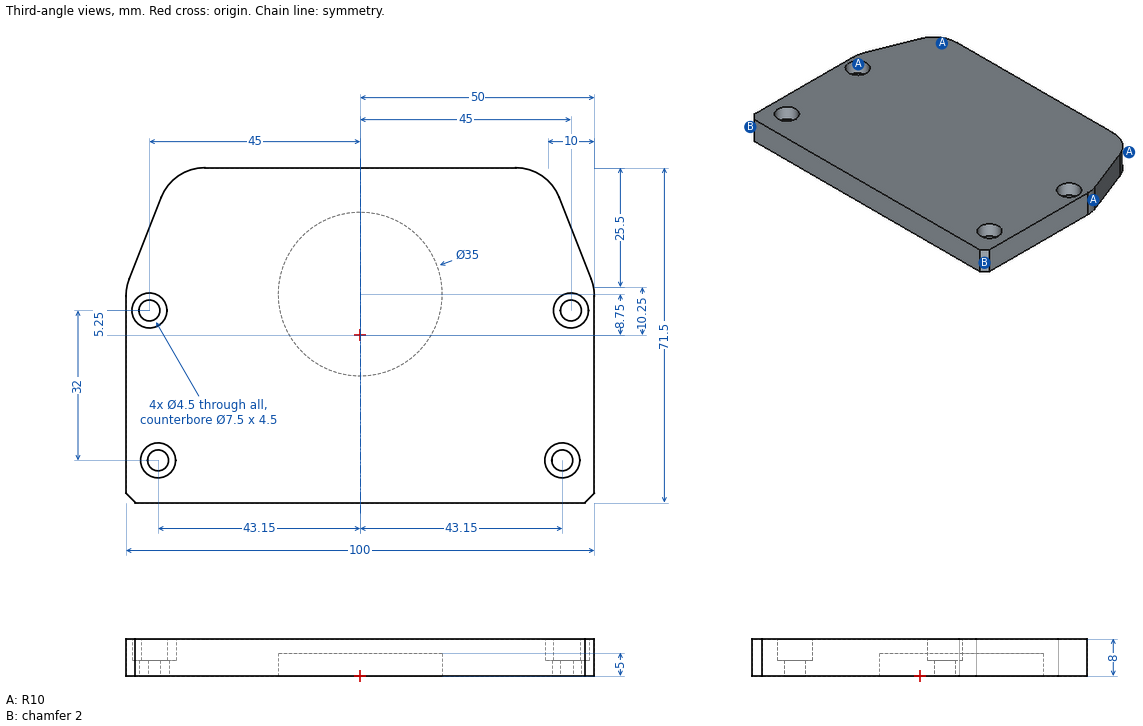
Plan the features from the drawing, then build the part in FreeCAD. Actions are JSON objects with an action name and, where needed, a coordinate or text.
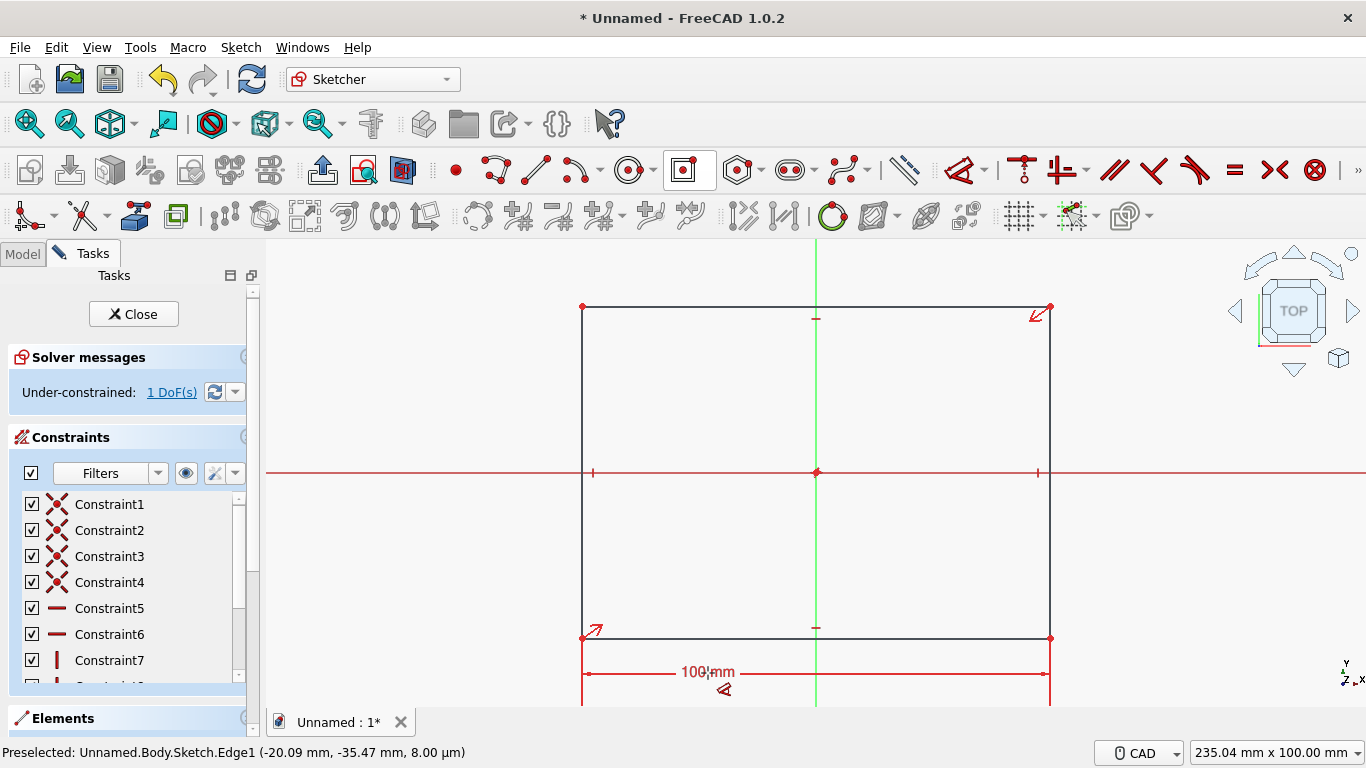
{"action": "left_click", "coordinate": [1050, 539]}
{"action": "left_click", "coordinate": [1084, 397]}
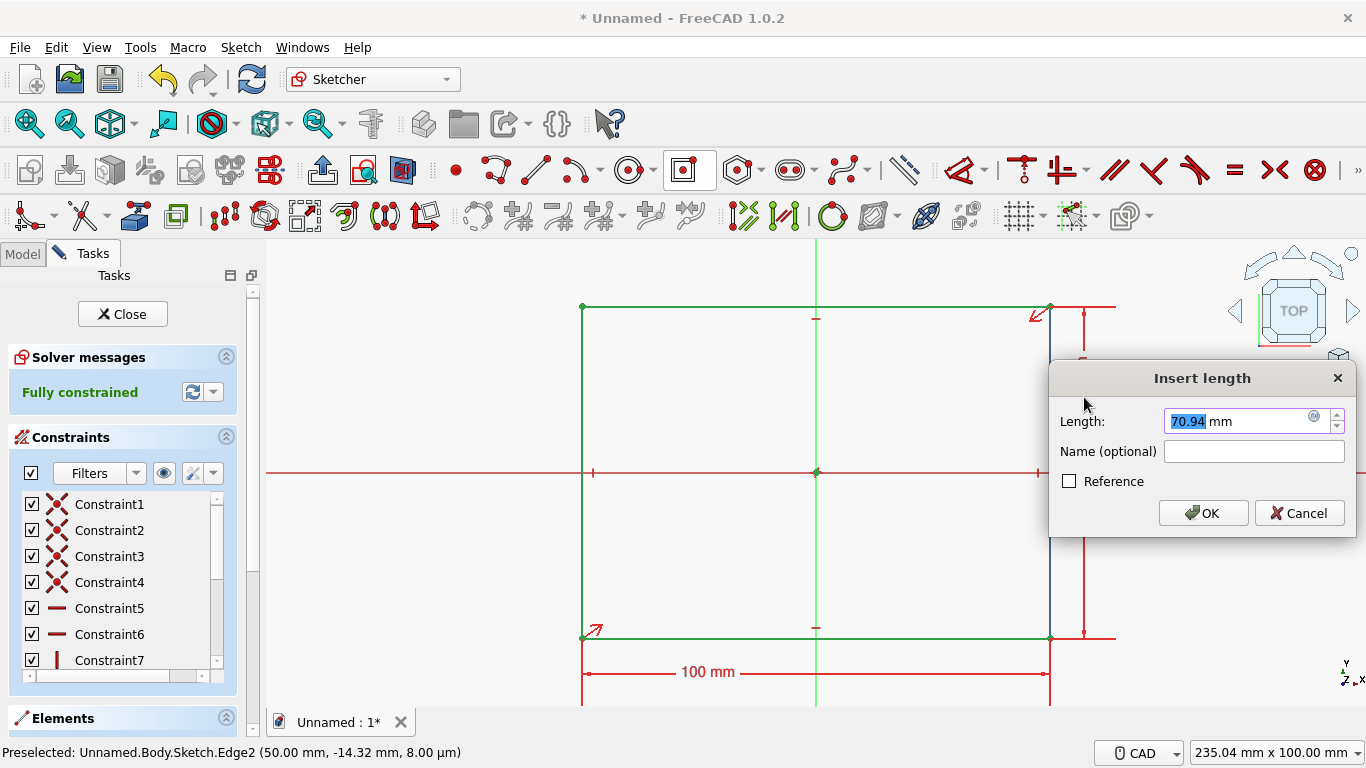
{"action": "type", "text": "71.5"}
{"action": "key", "text": "Return"}
{"action": "key", "text": "Escape"}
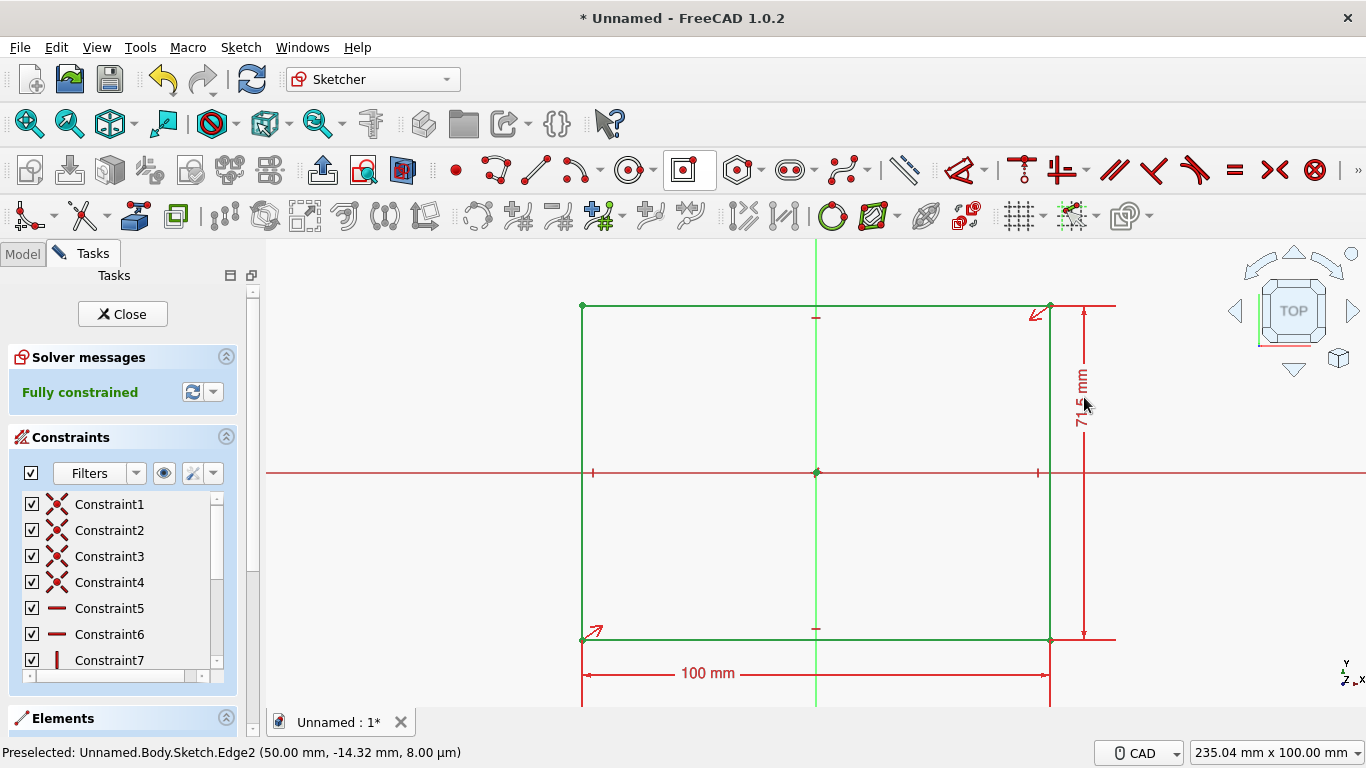
{"action": "left_click", "coordinate": [123, 314]}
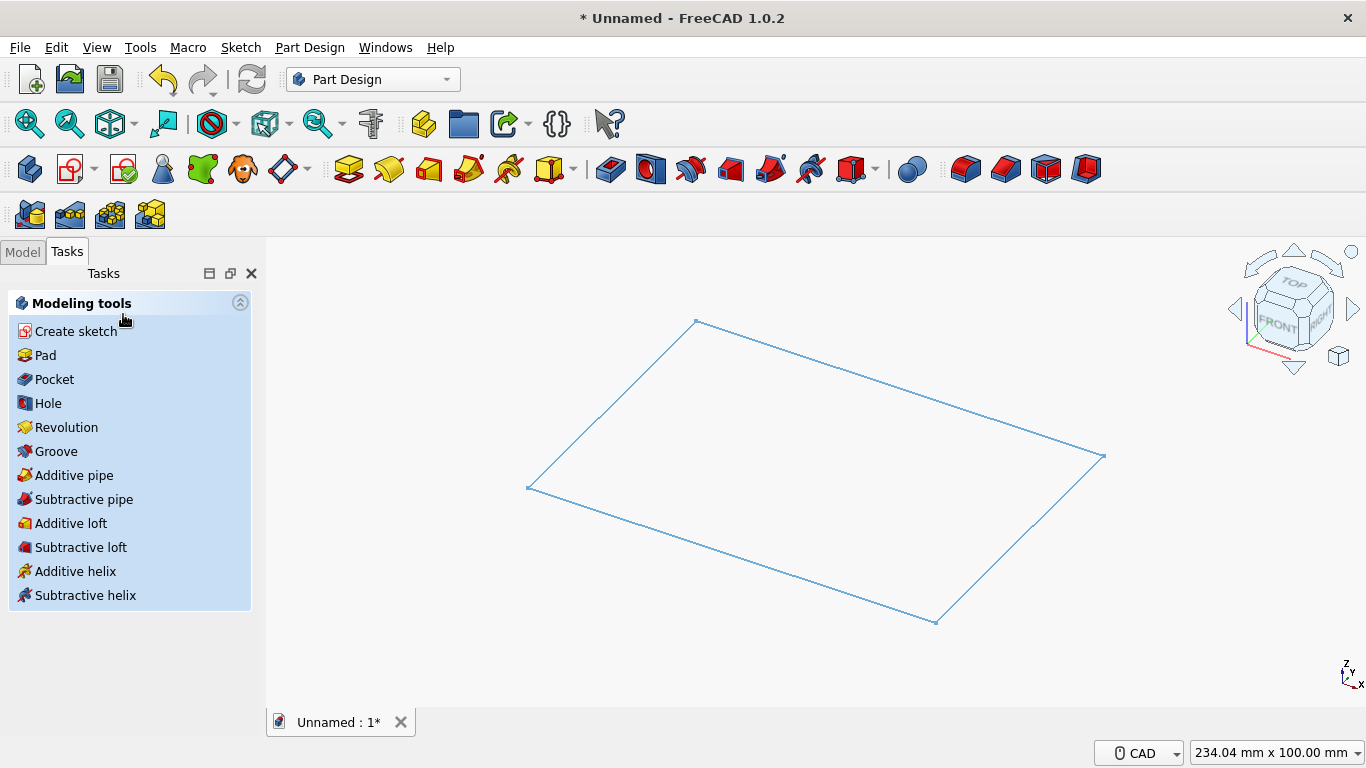
{"action": "left_click", "coordinate": [350, 170]}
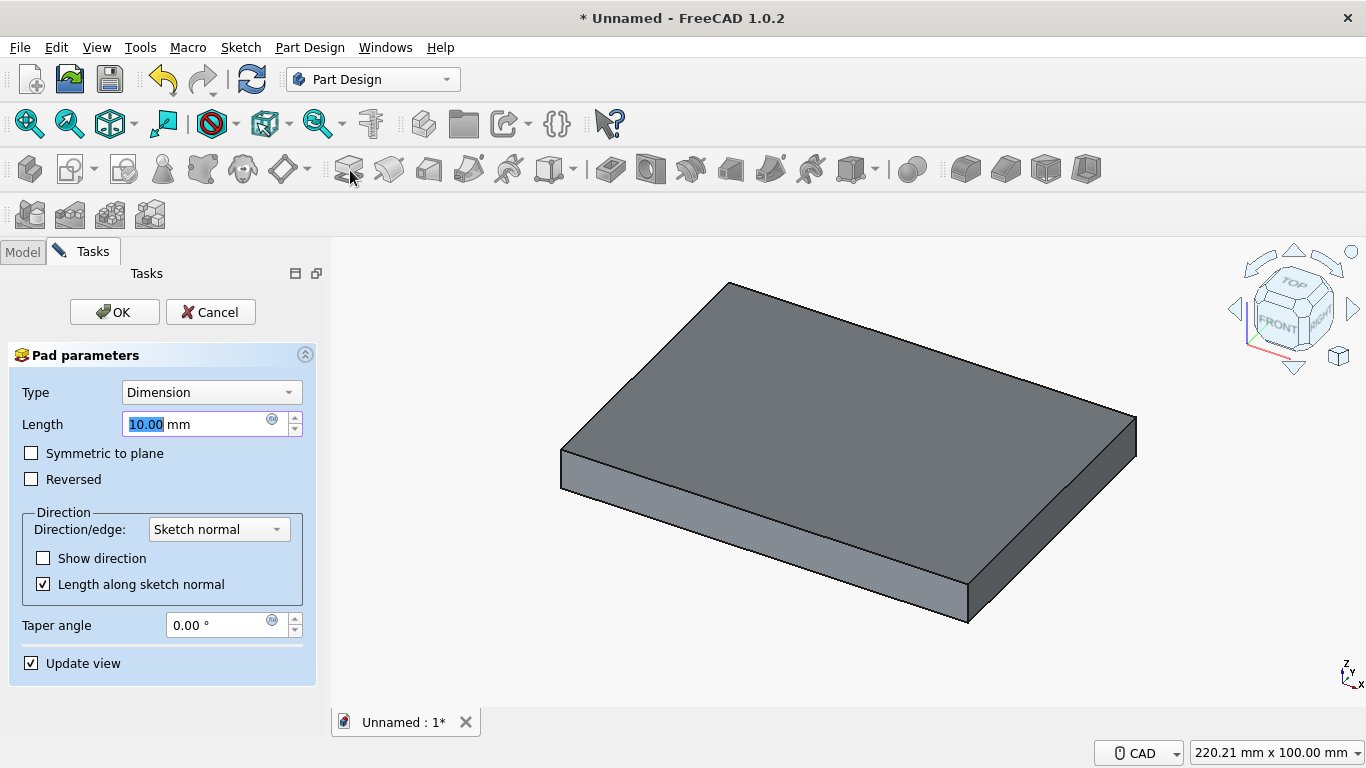
{"action": "type", "text": "8"}
{"action": "key", "text": "Tab"}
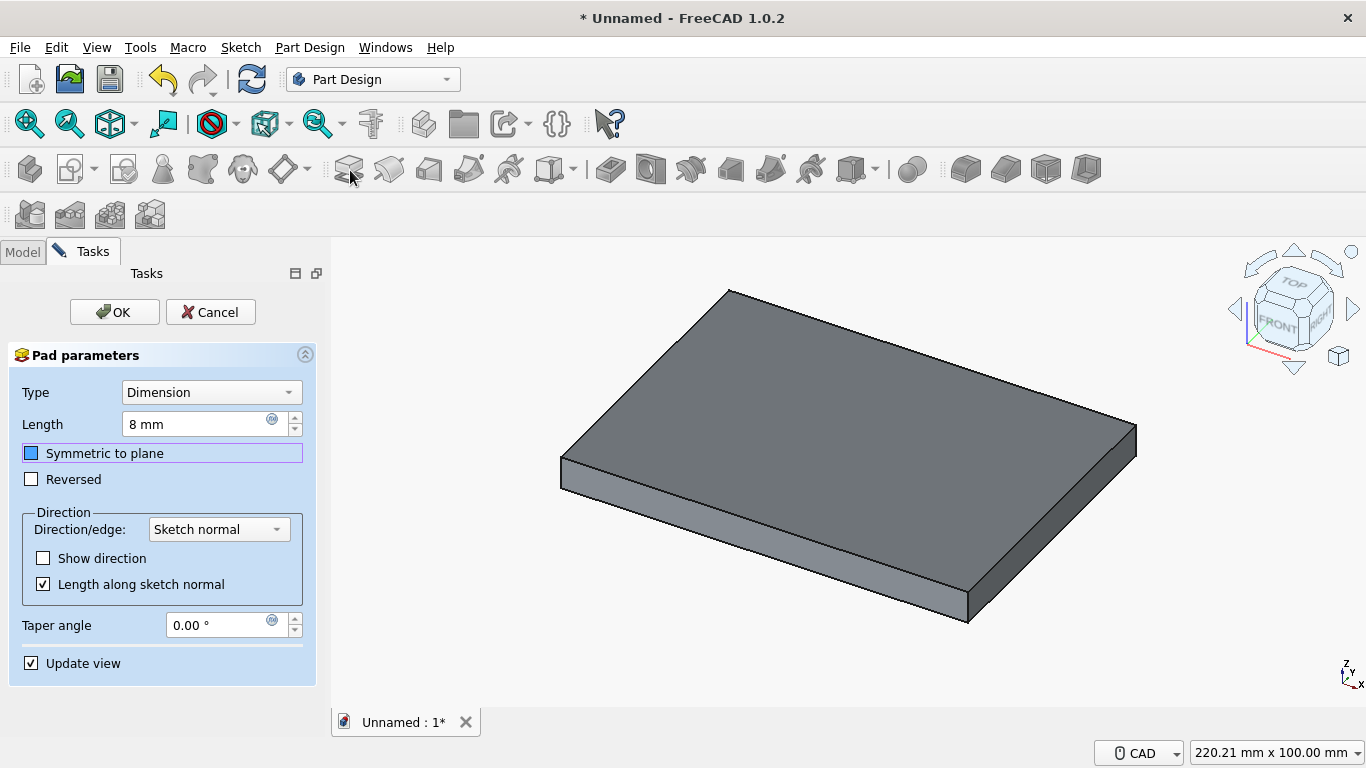
{"action": "left_click", "coordinate": [115, 312]}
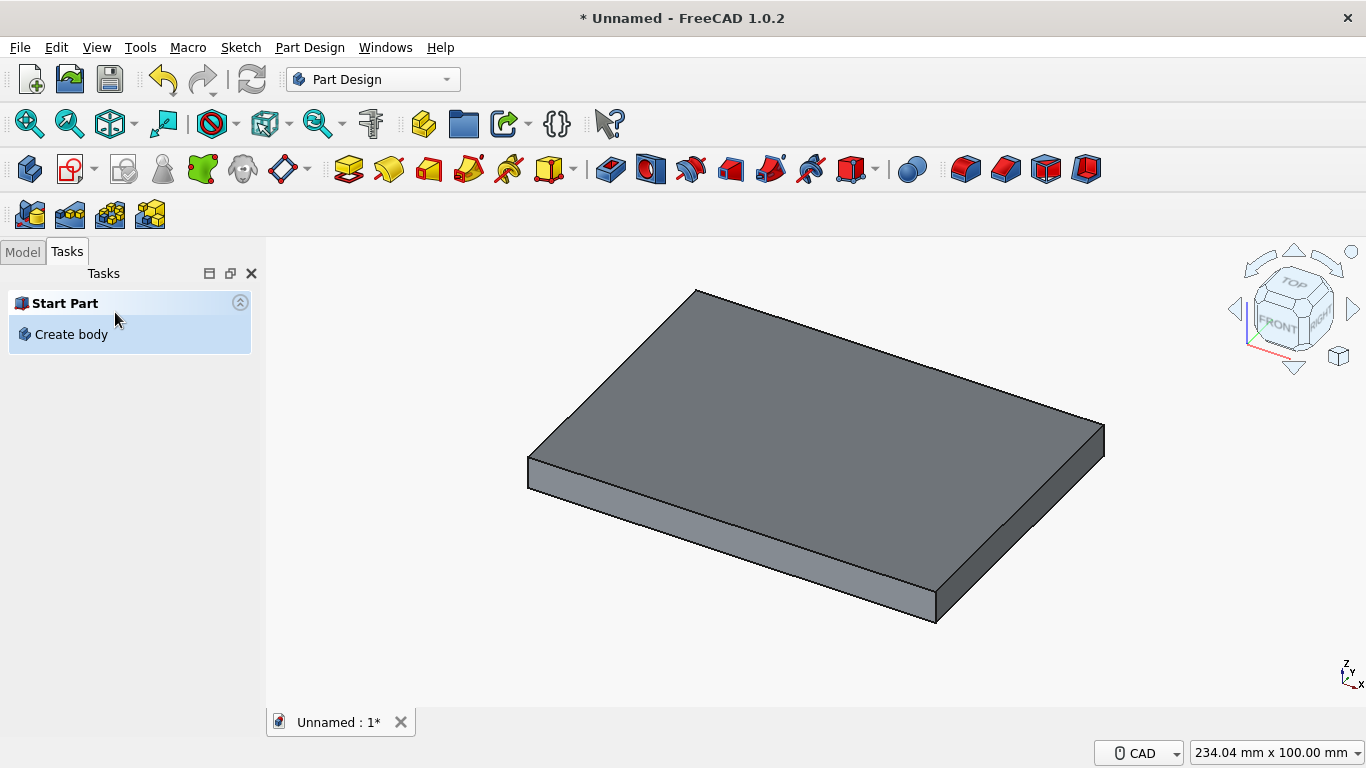
{"action": "key", "text": "5"}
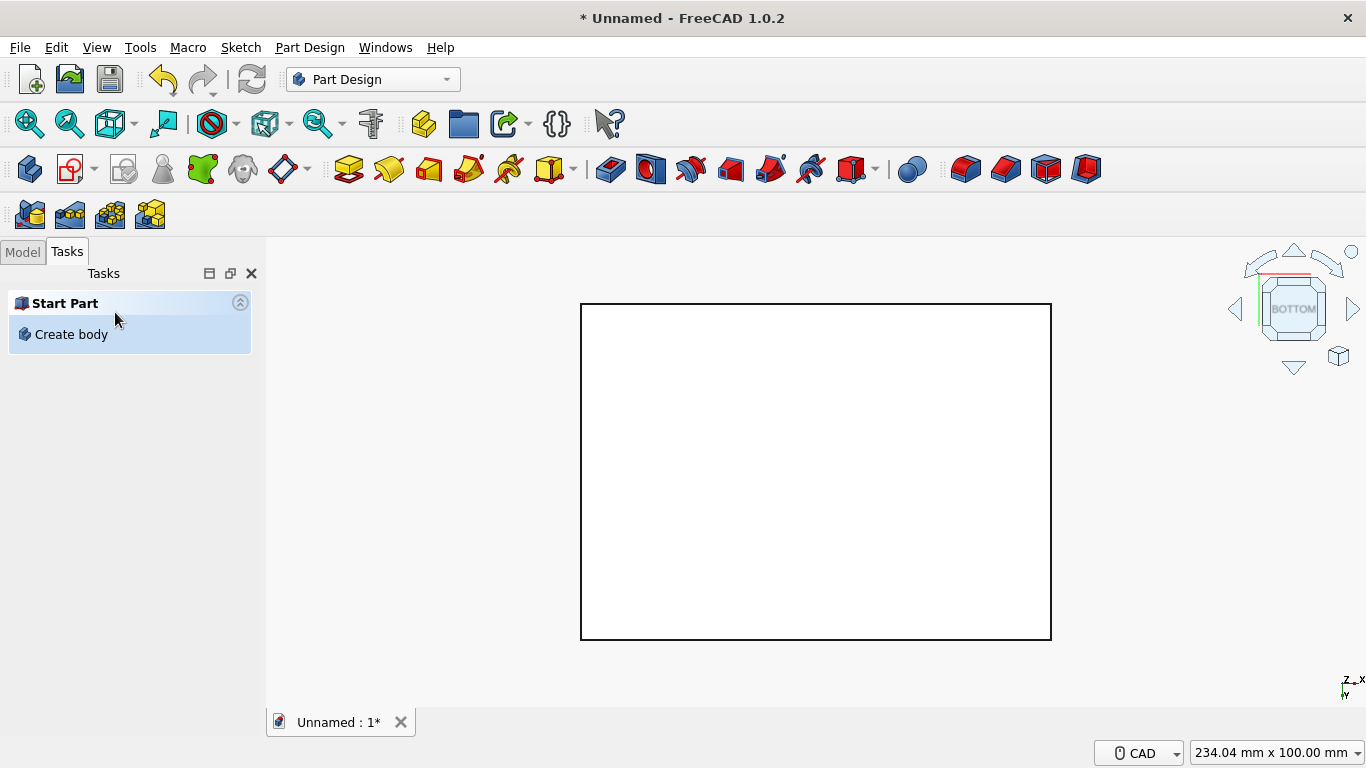
{"action": "left_click", "coordinate": [816, 471]}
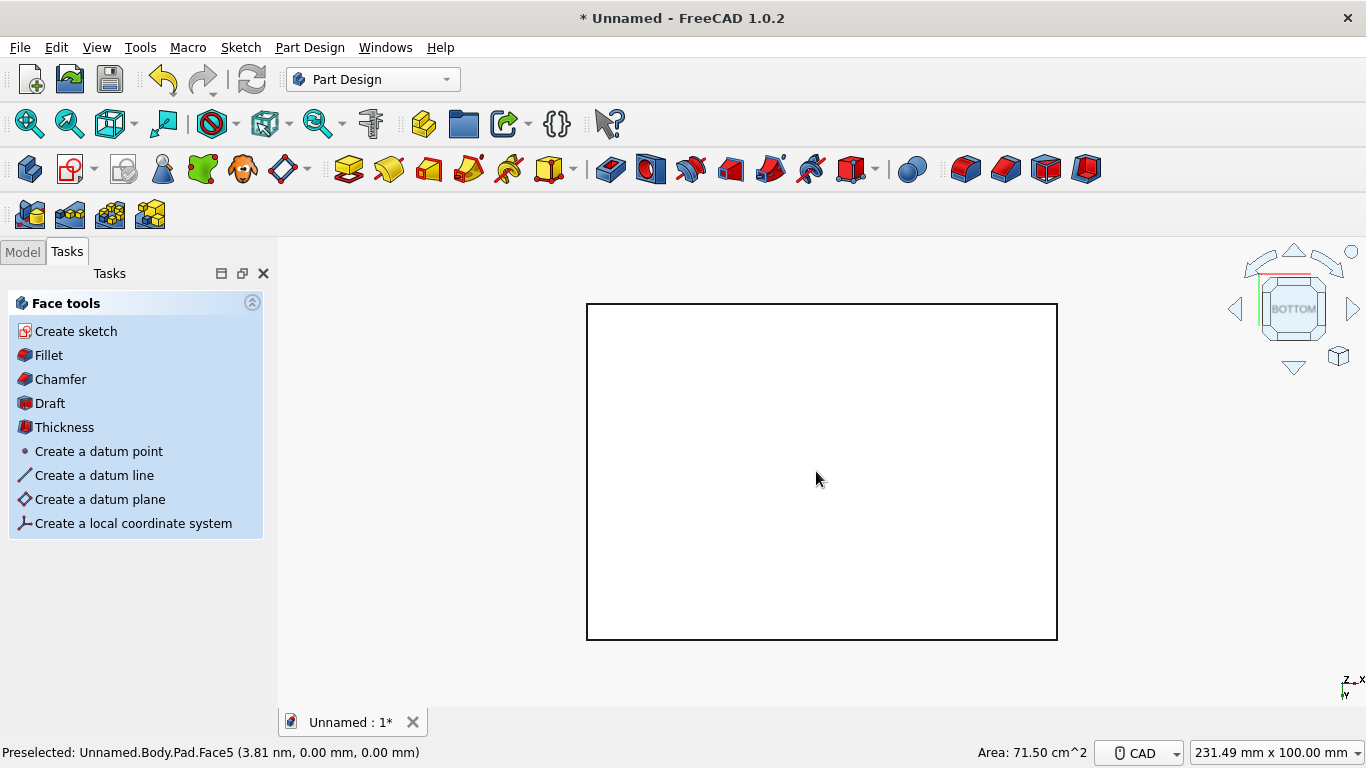
{"action": "left_click", "coordinate": [70, 170]}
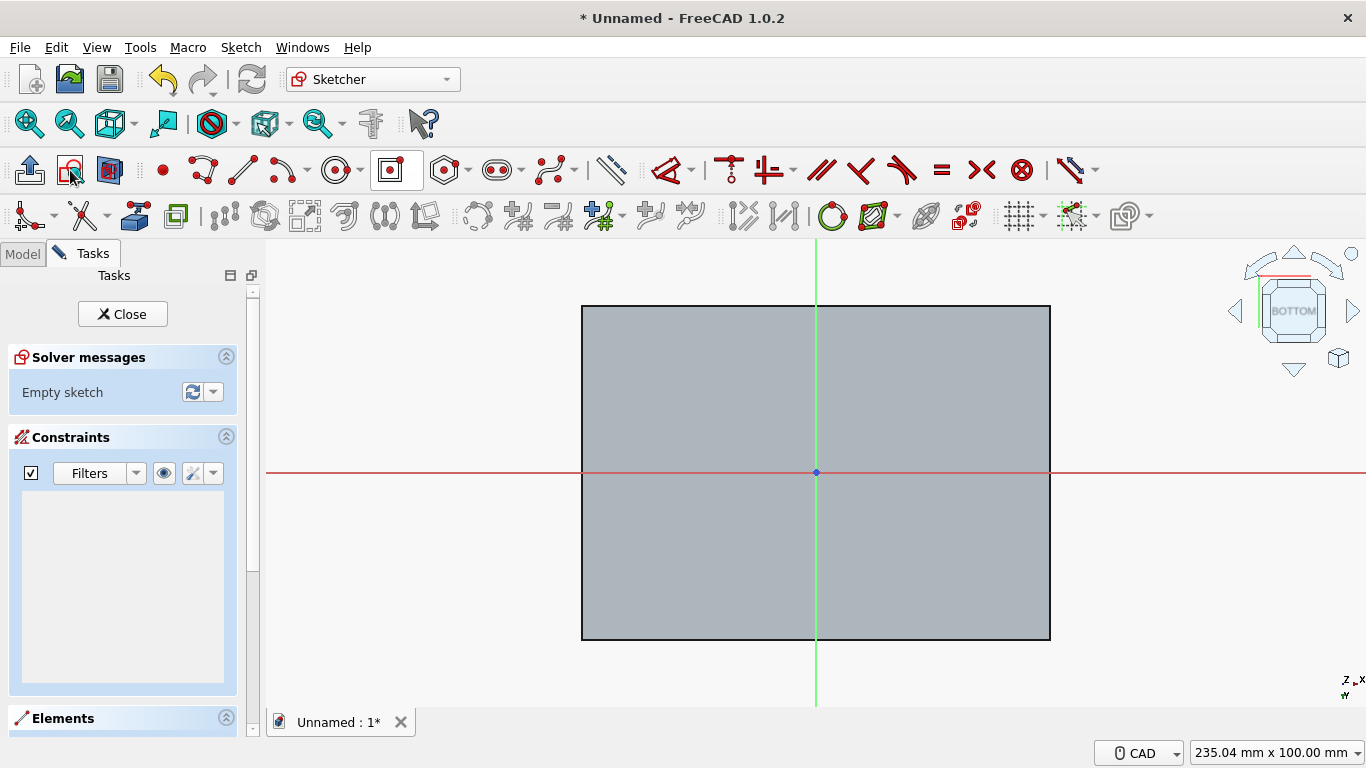
{"action": "scroll", "coordinate": [955, 679], "scroll_direction": "up", "scroll_amount": 2}